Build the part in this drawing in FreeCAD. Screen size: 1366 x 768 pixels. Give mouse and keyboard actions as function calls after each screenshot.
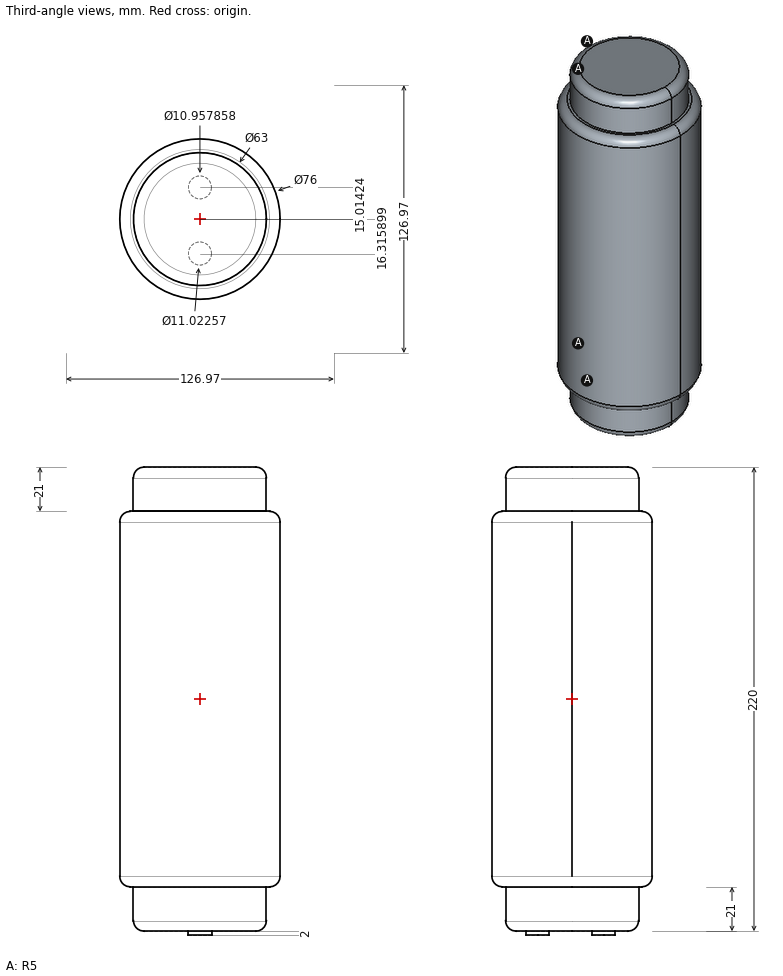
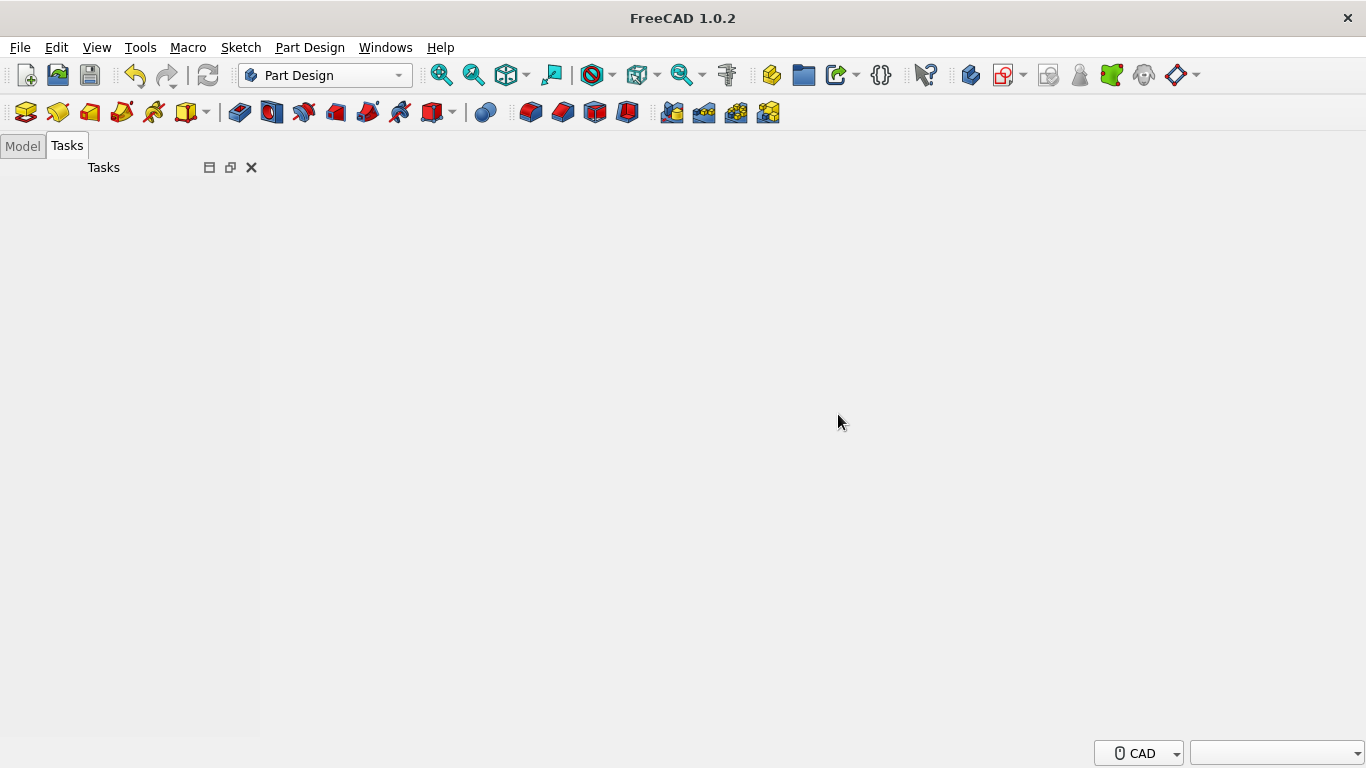
click(26, 76)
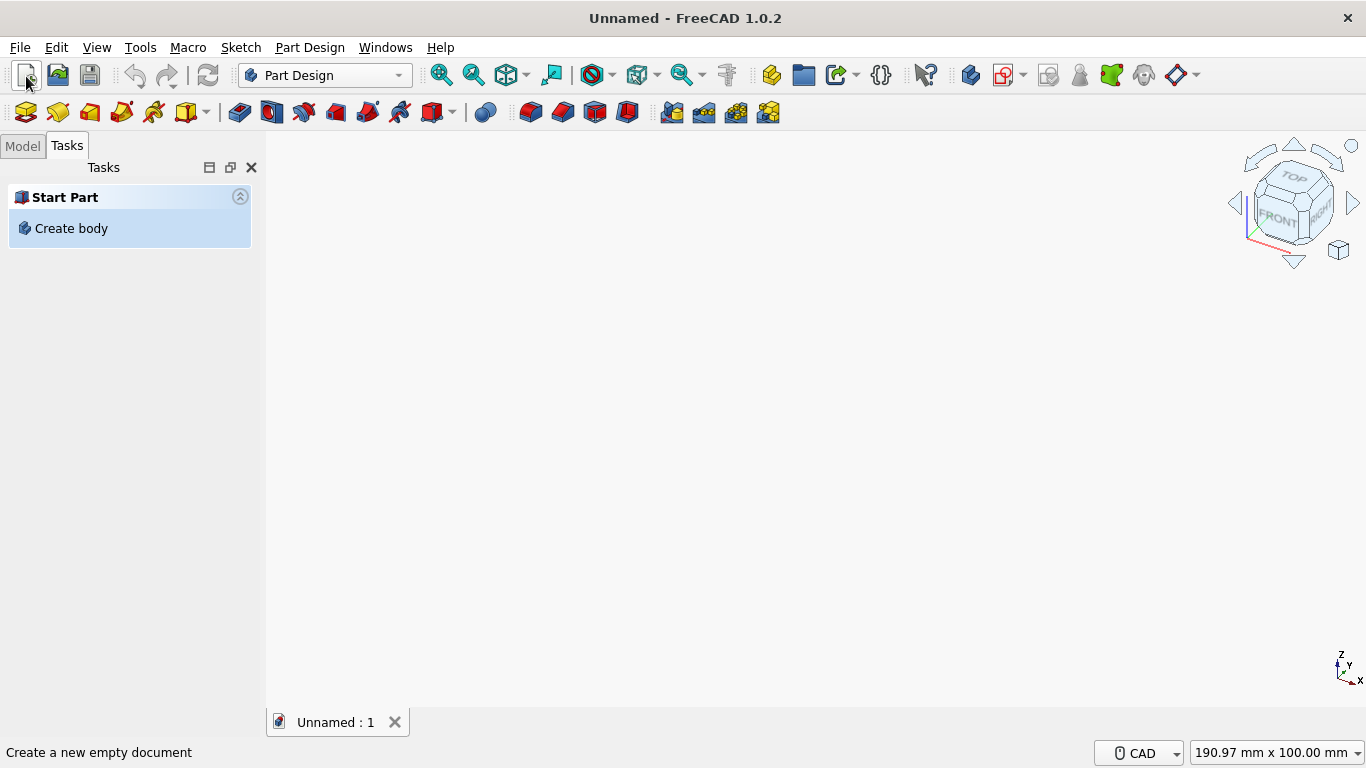
click(1004, 76)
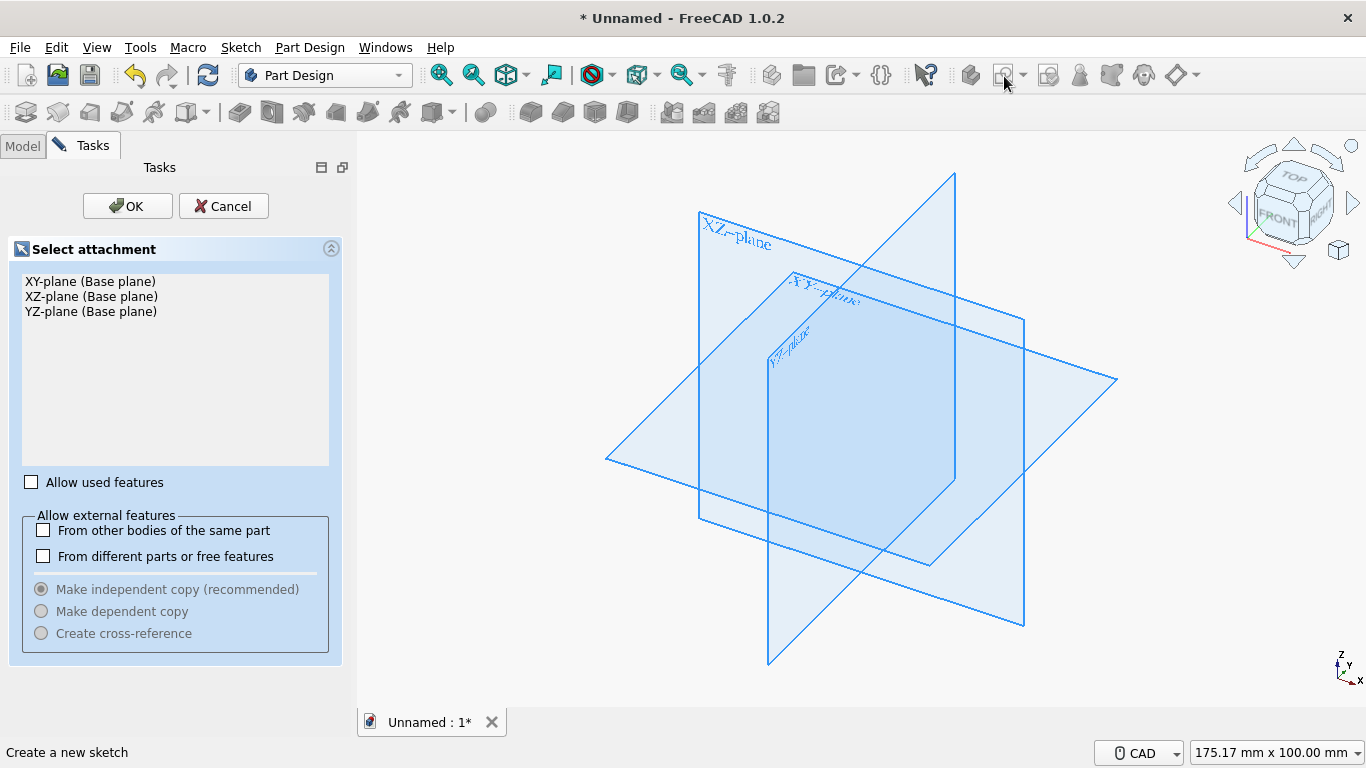
click(82, 282)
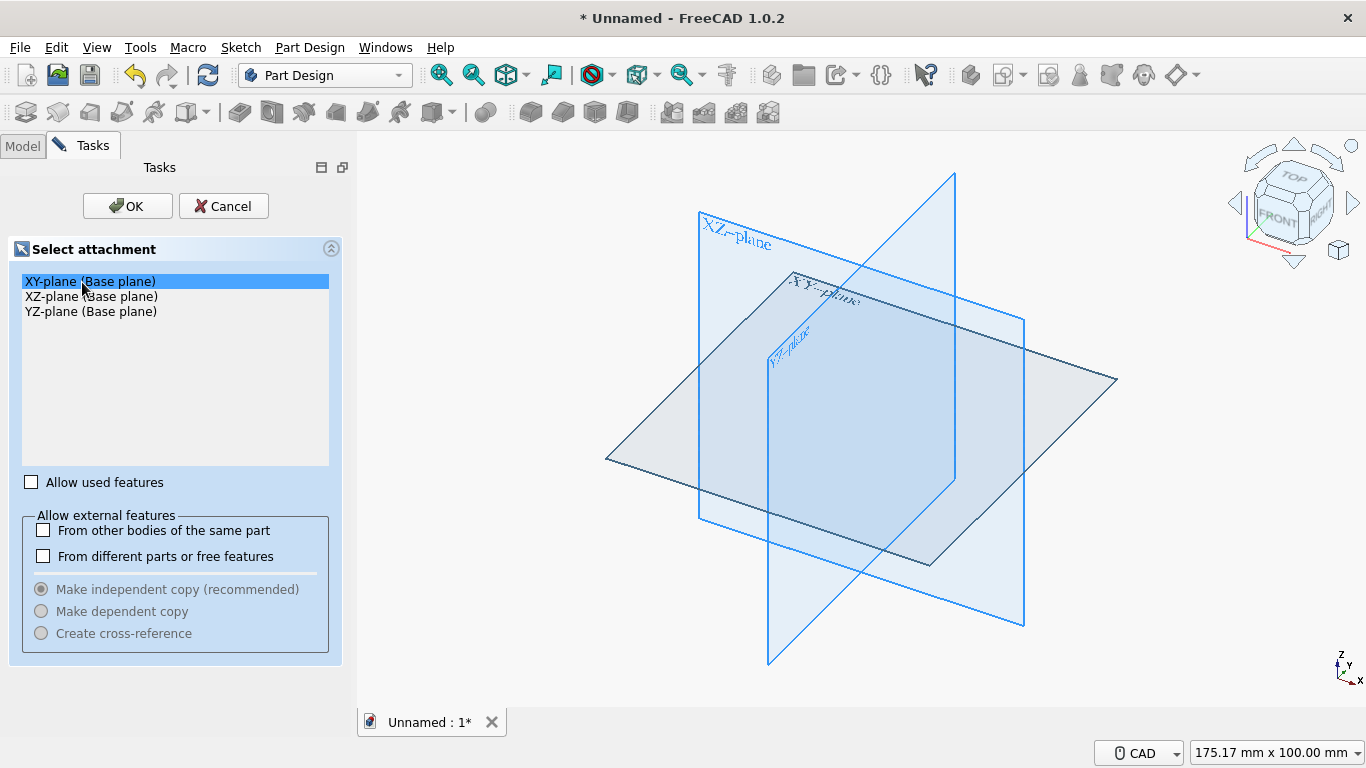
click(128, 206)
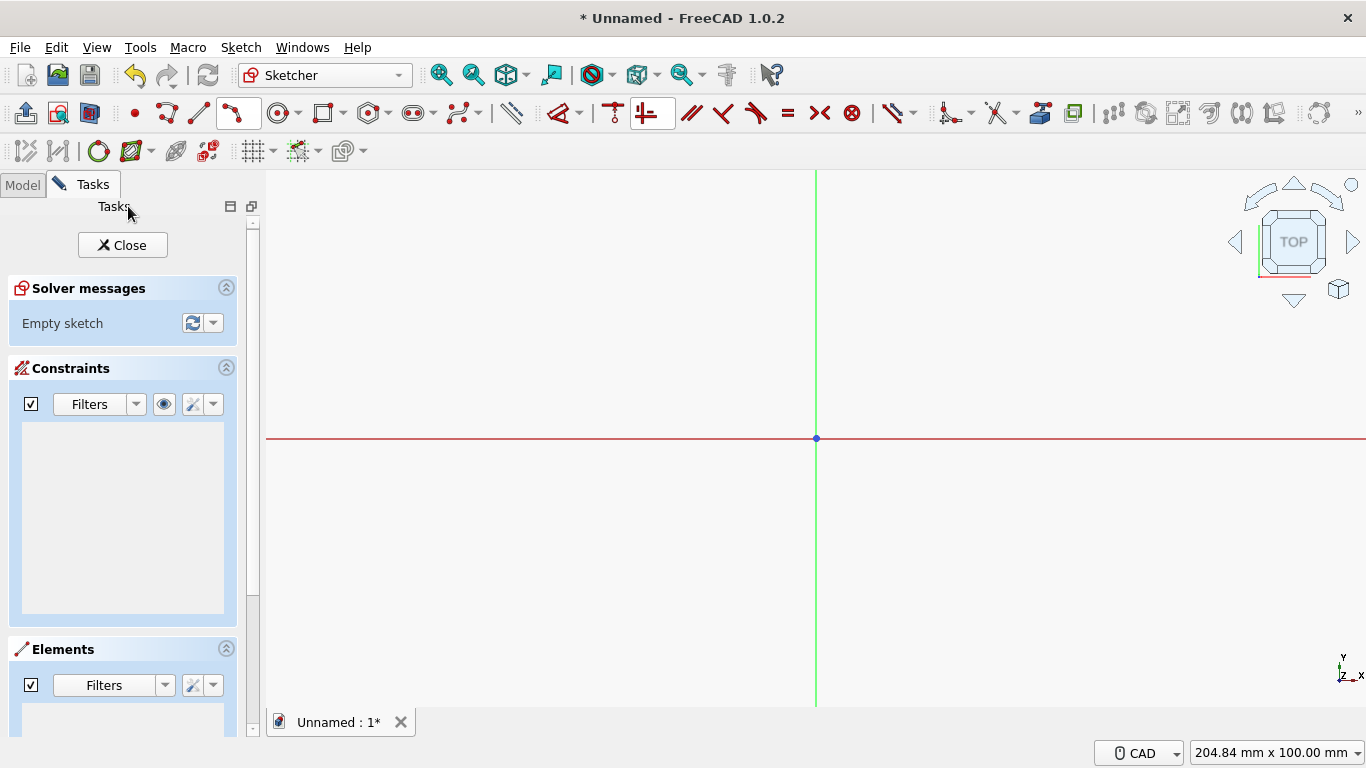
click(278, 114)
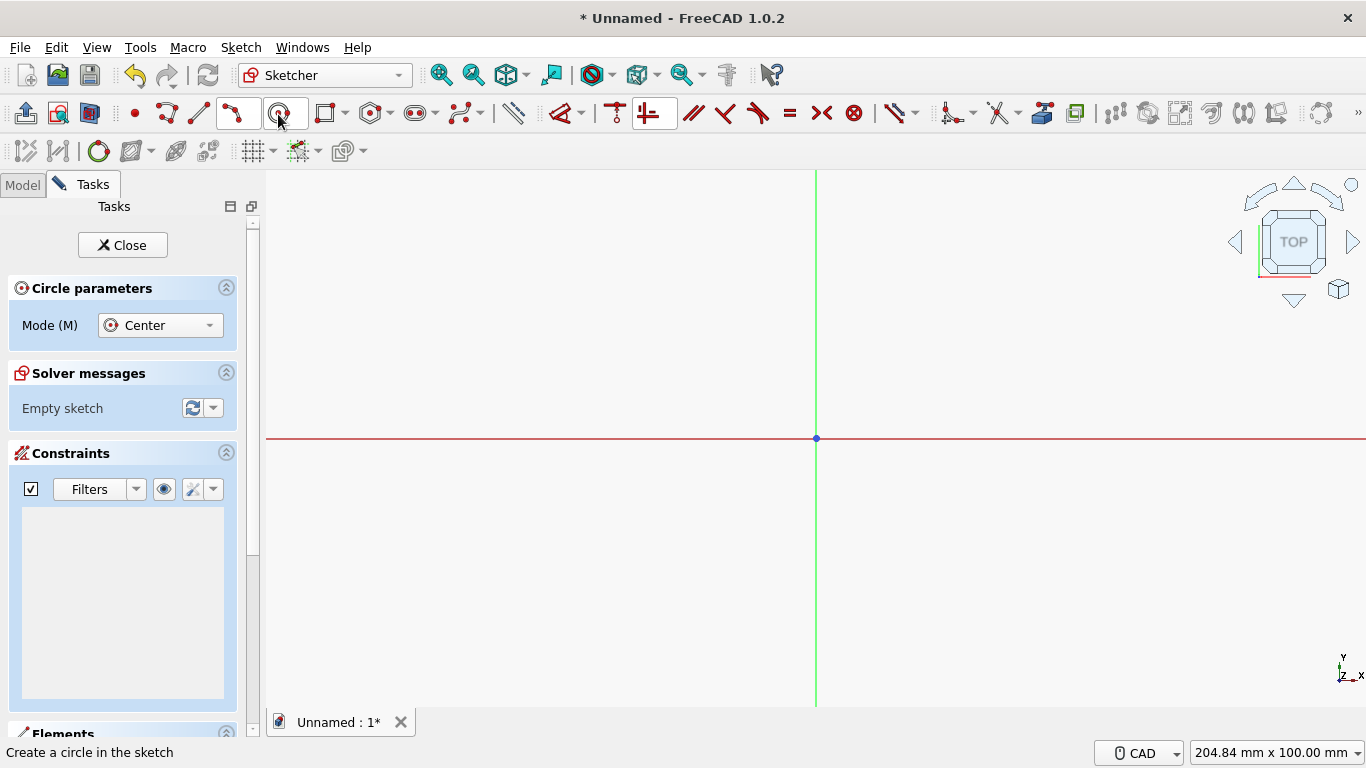
click(816, 438)
move(960, 294)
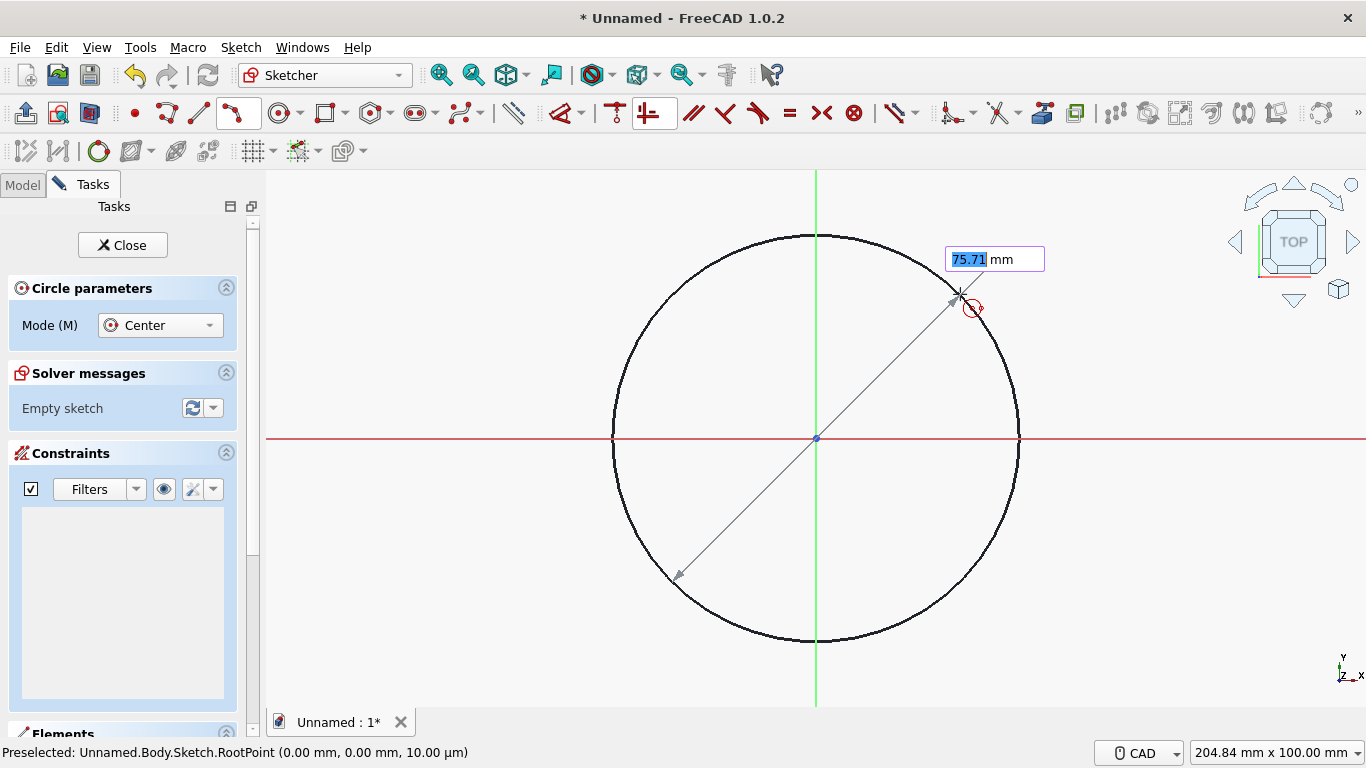
text(76)
key(Return)
key(Escape)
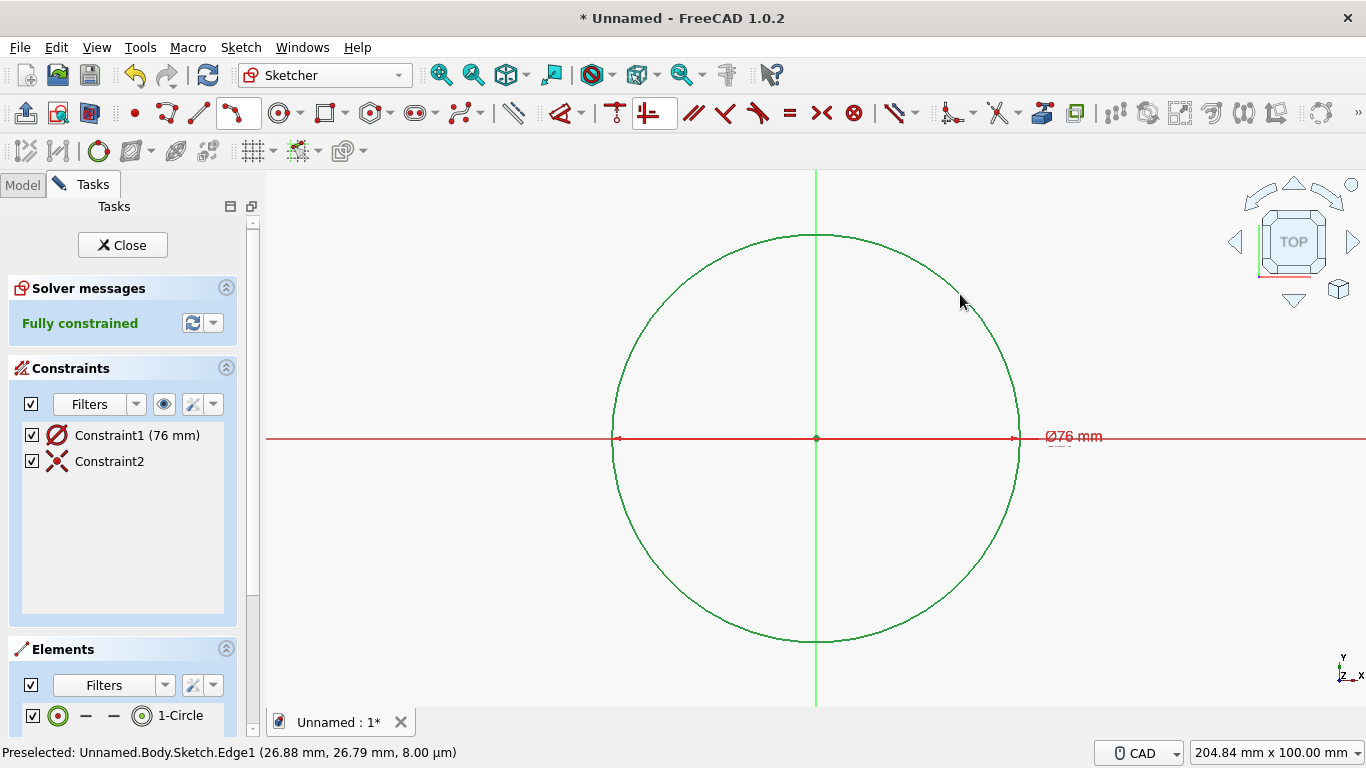
click(123, 245)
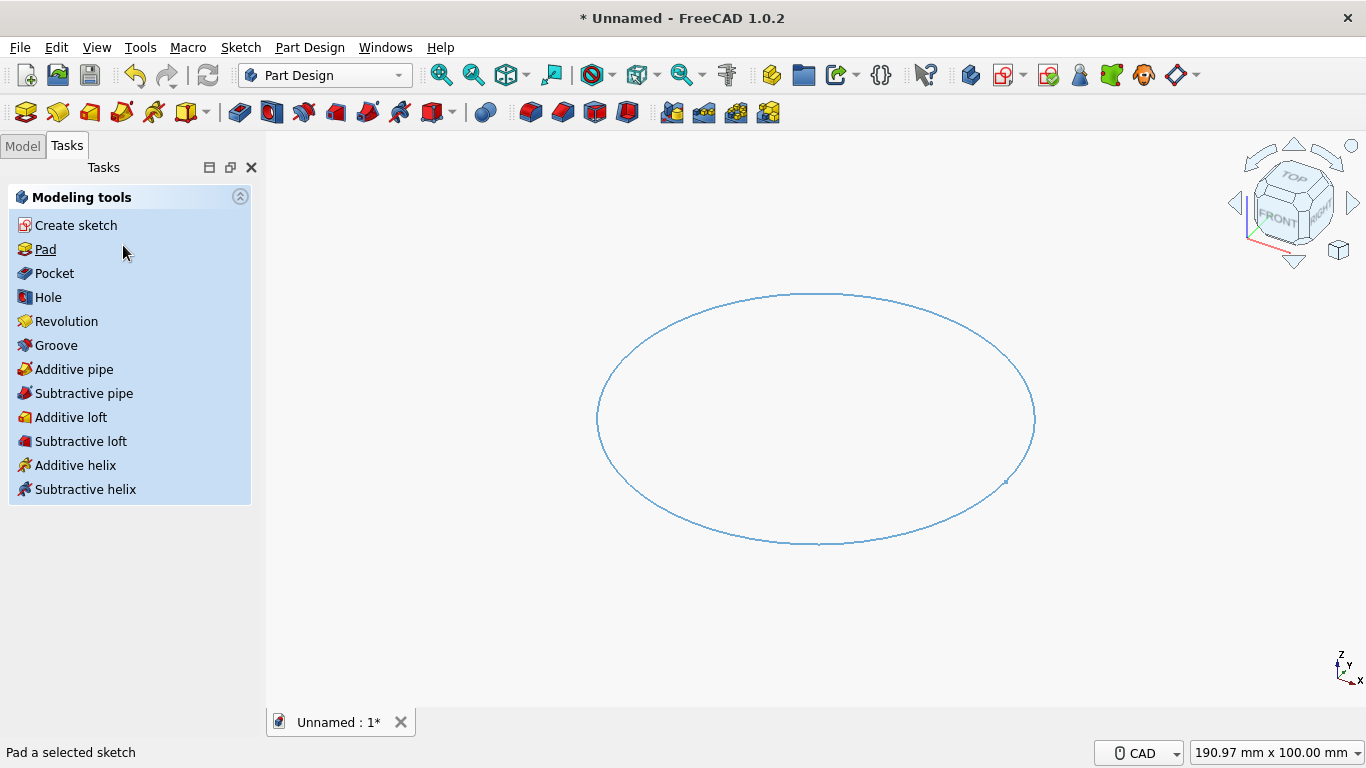
click(26, 112)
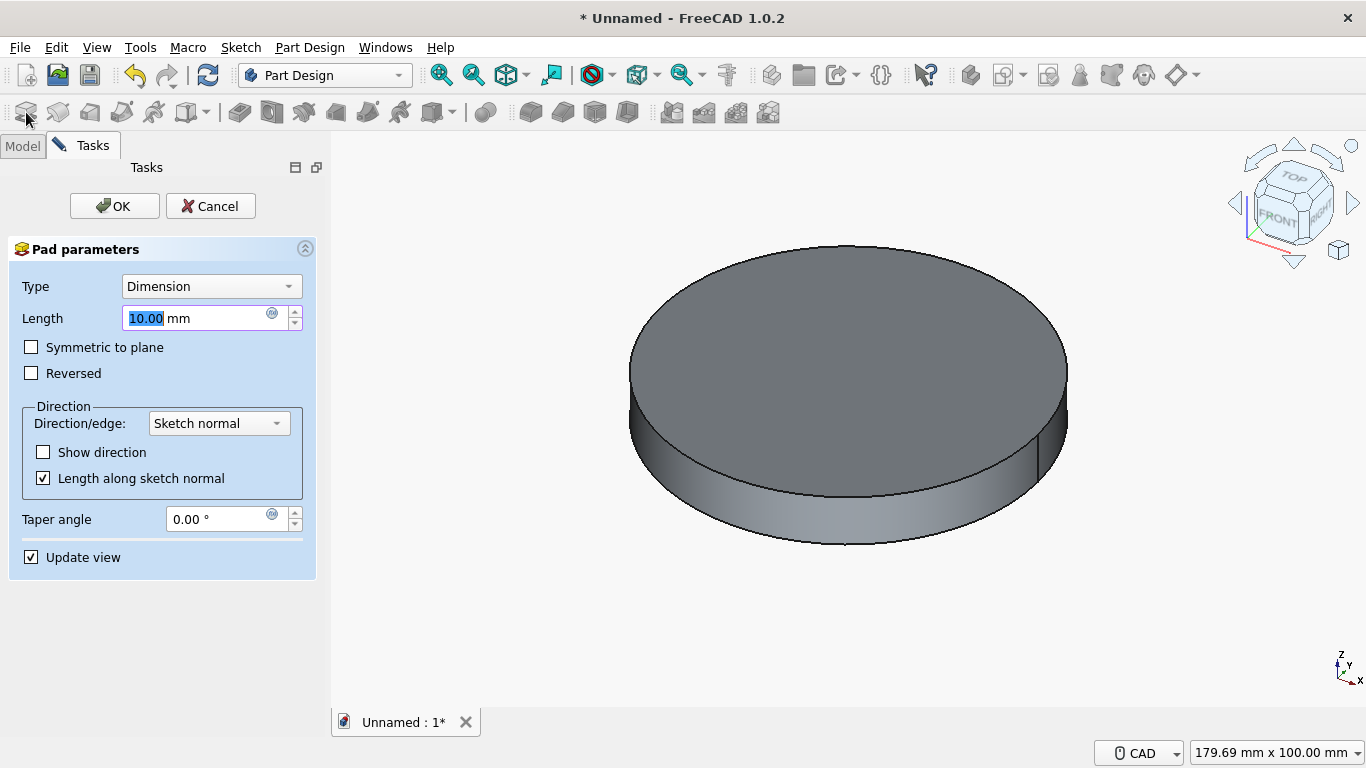
text(220)
key(Tab)